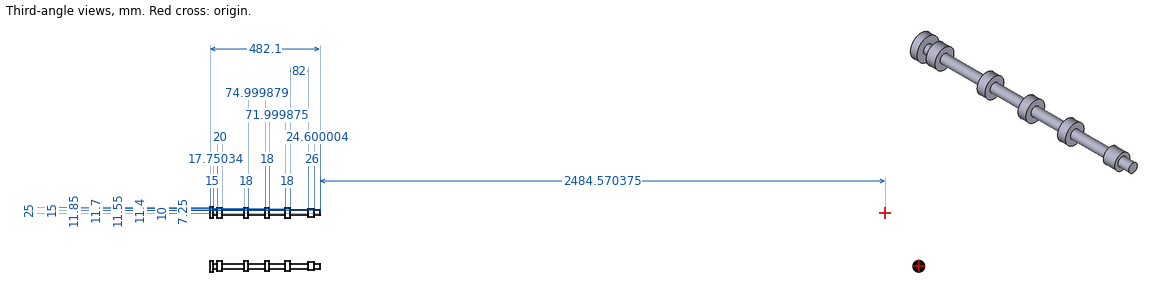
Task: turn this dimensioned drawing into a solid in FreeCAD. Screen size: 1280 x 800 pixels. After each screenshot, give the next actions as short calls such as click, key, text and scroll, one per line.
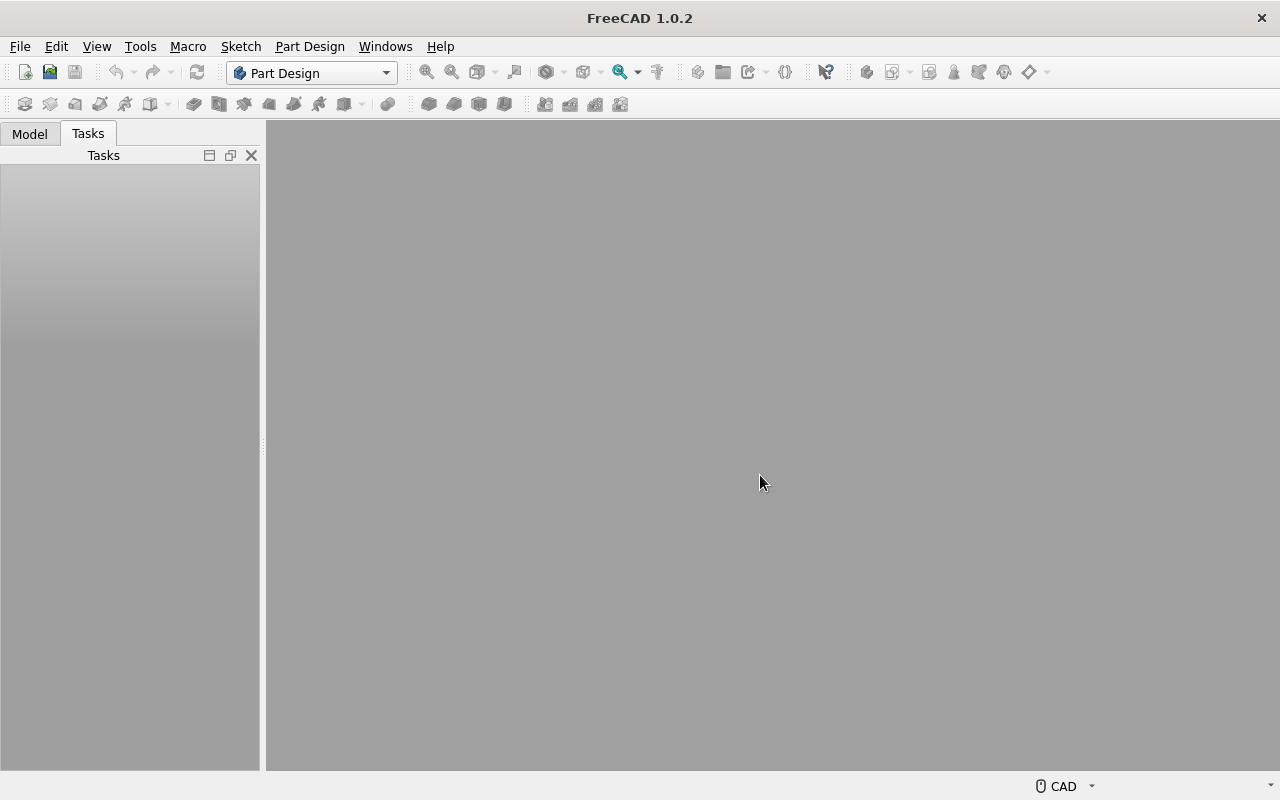
click(25, 72)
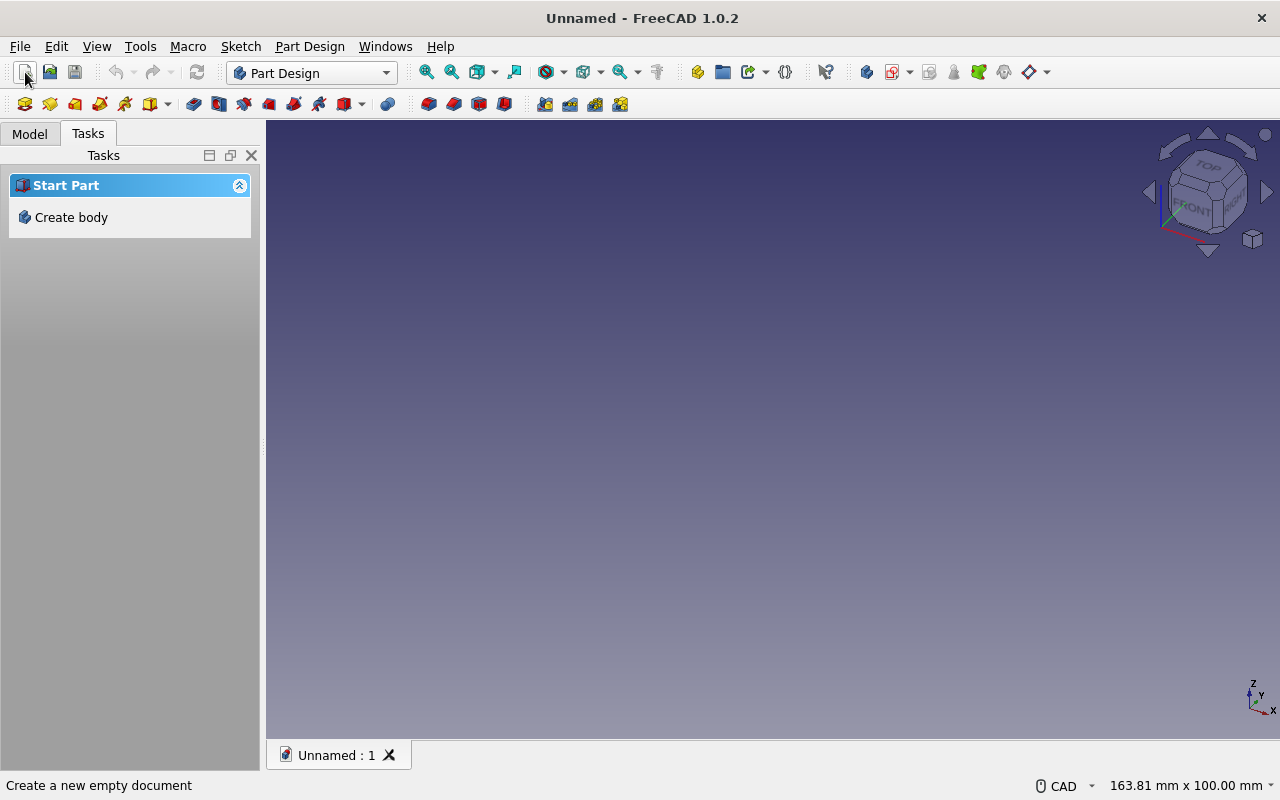
click(892, 72)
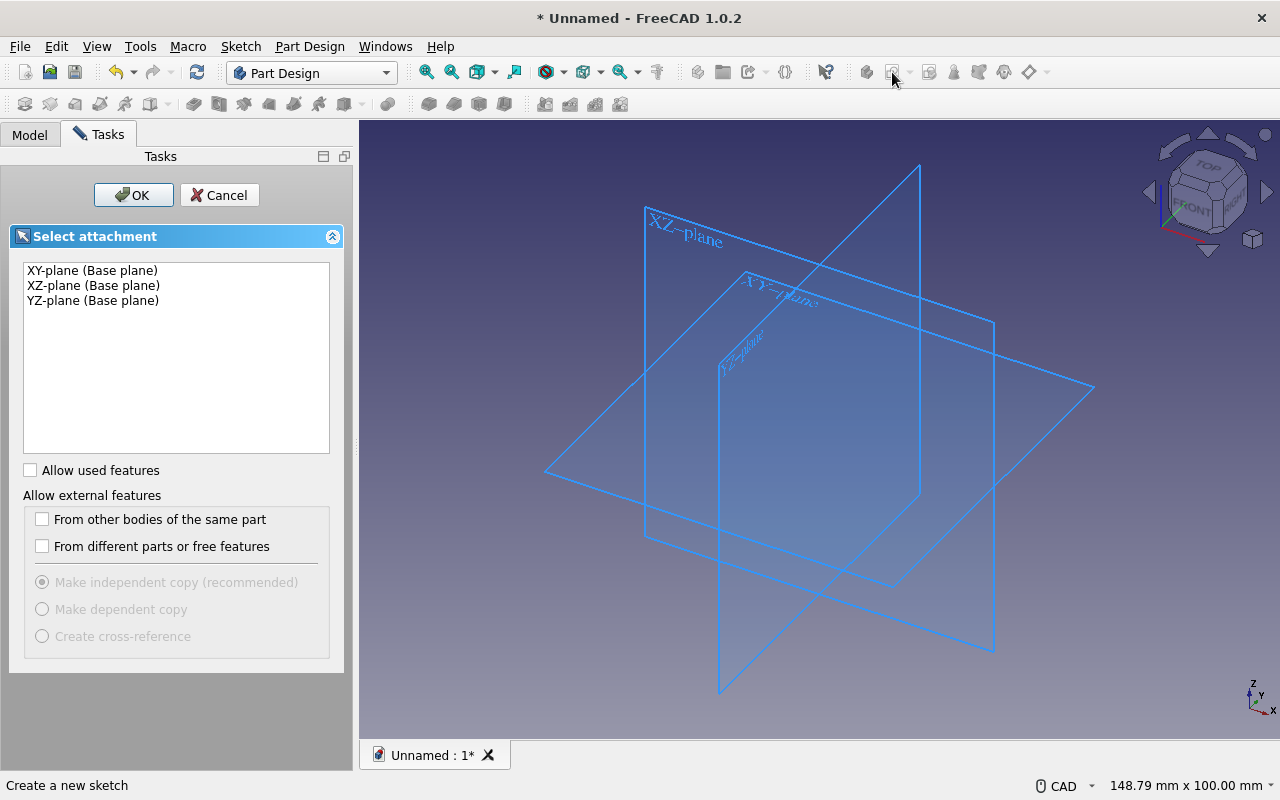
click(84, 270)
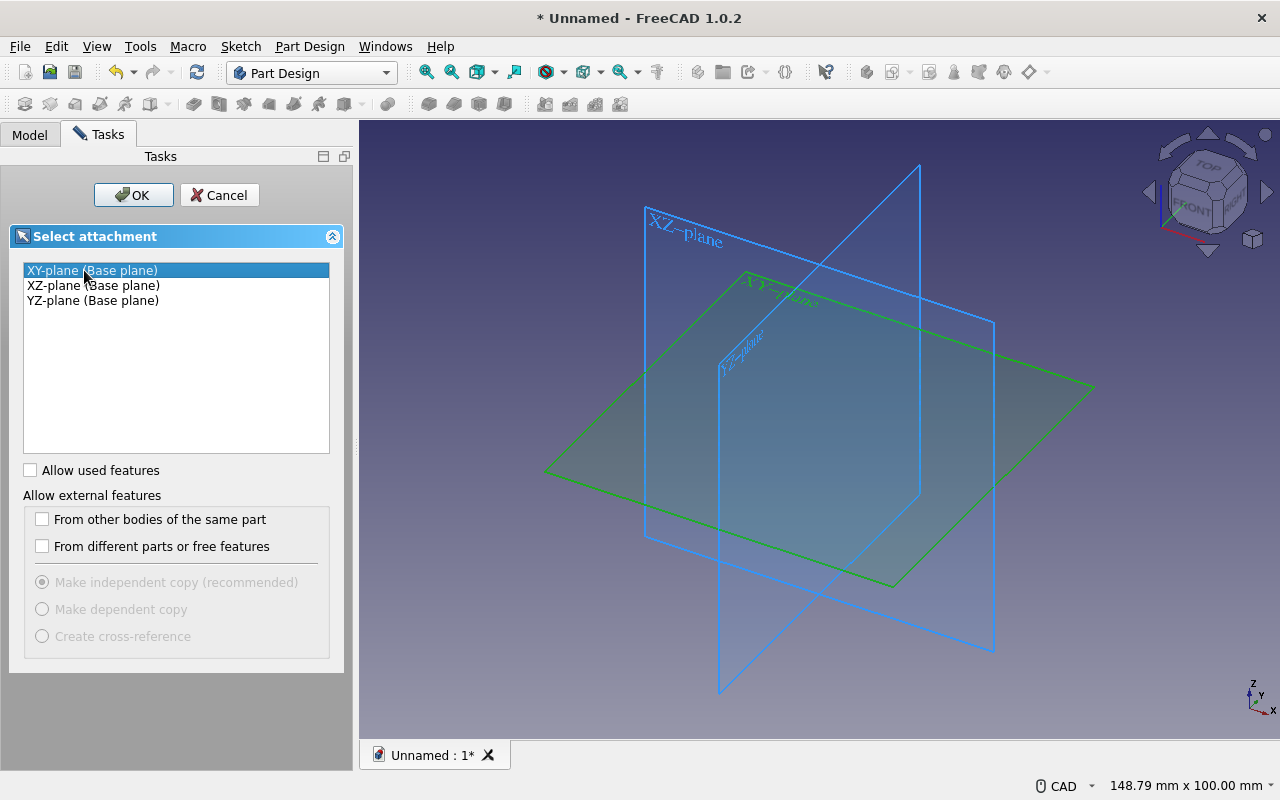
click(134, 195)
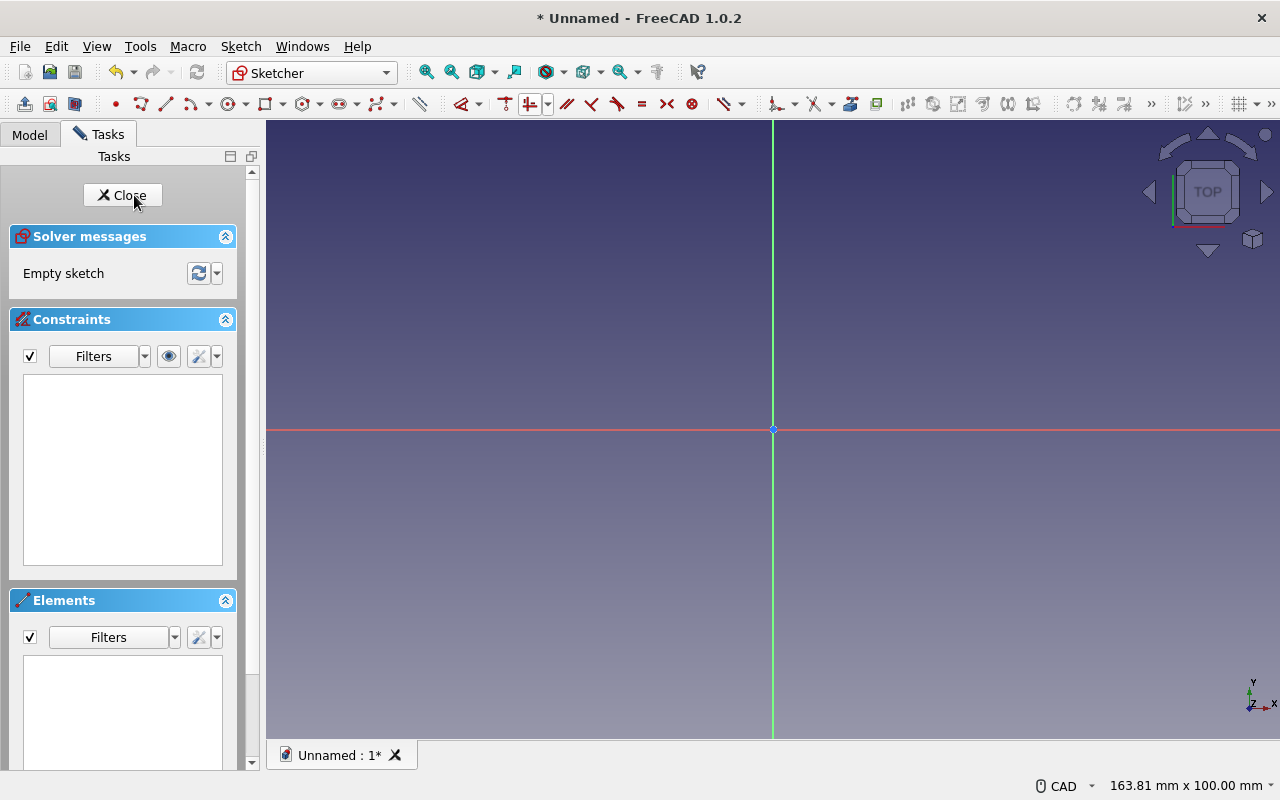
scroll(704, 430, down, 8)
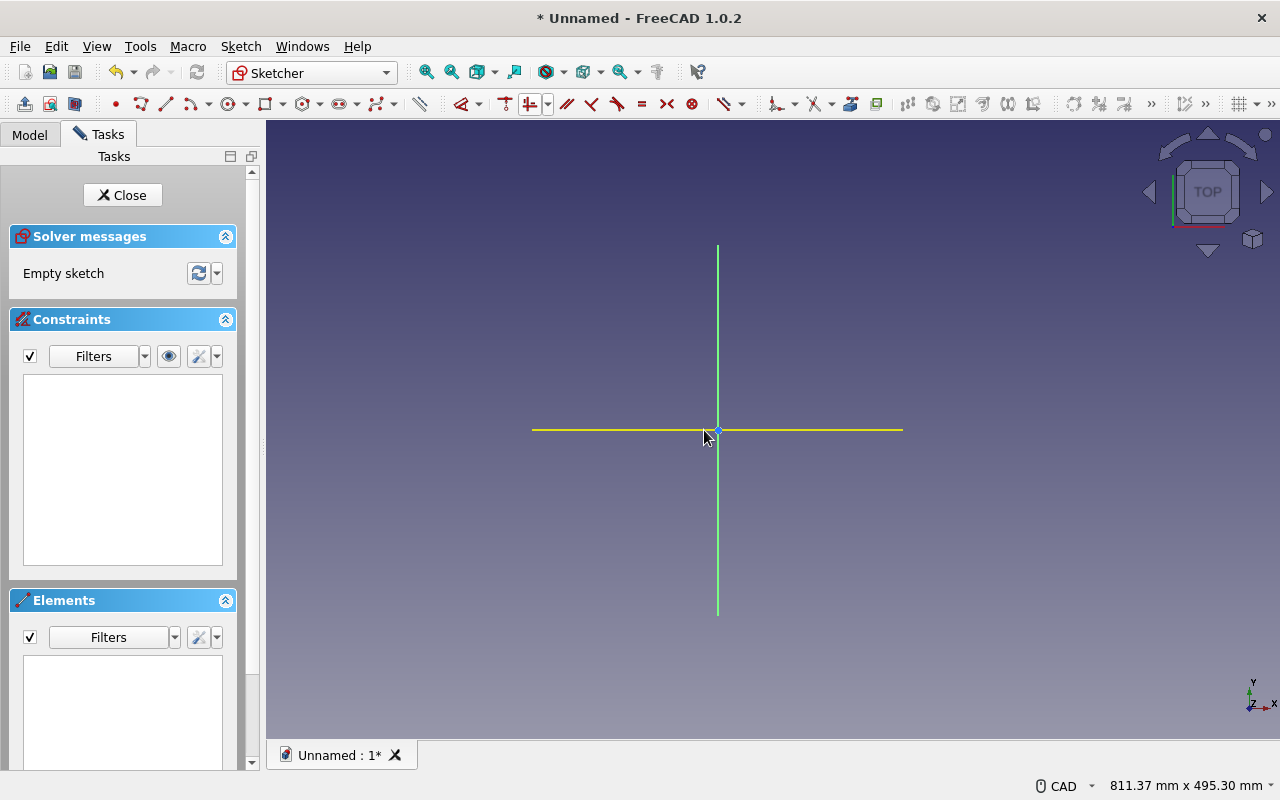
scroll(704, 430, down, 5)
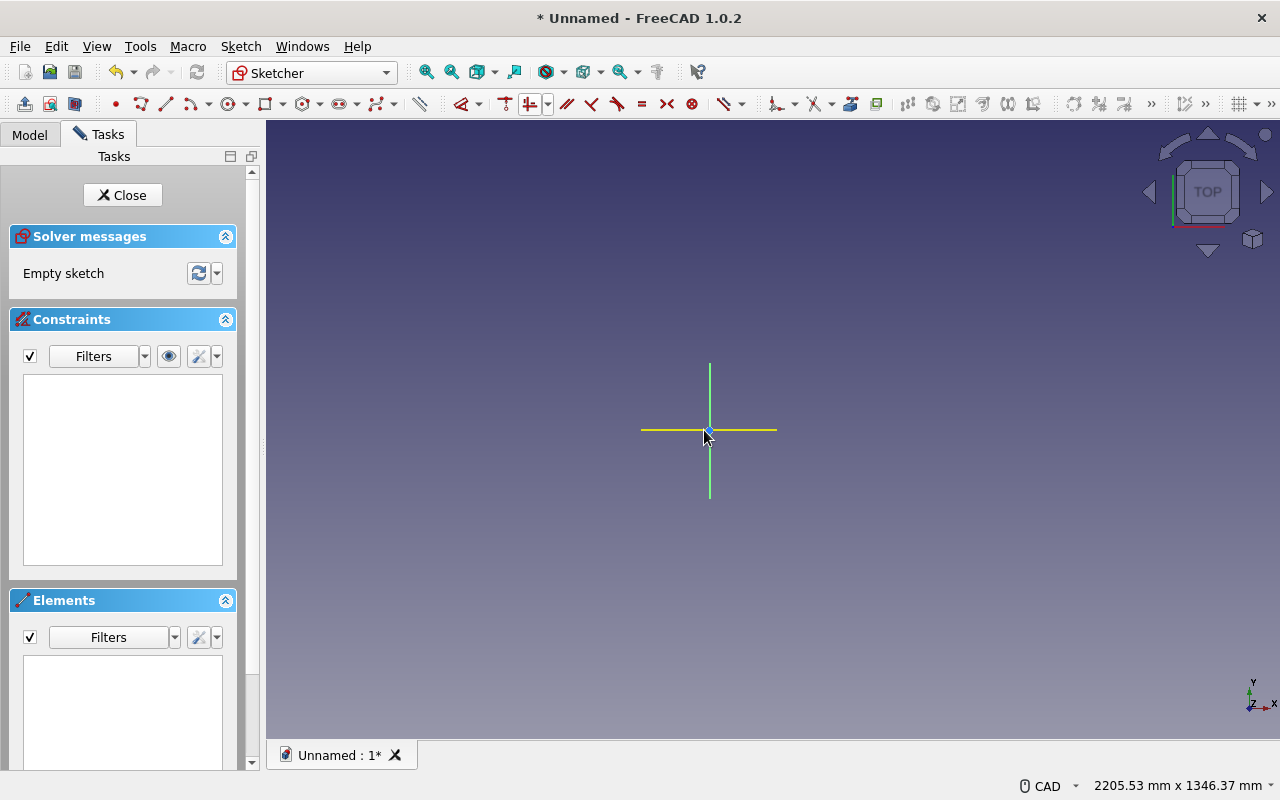
scroll(704, 430, down, 5)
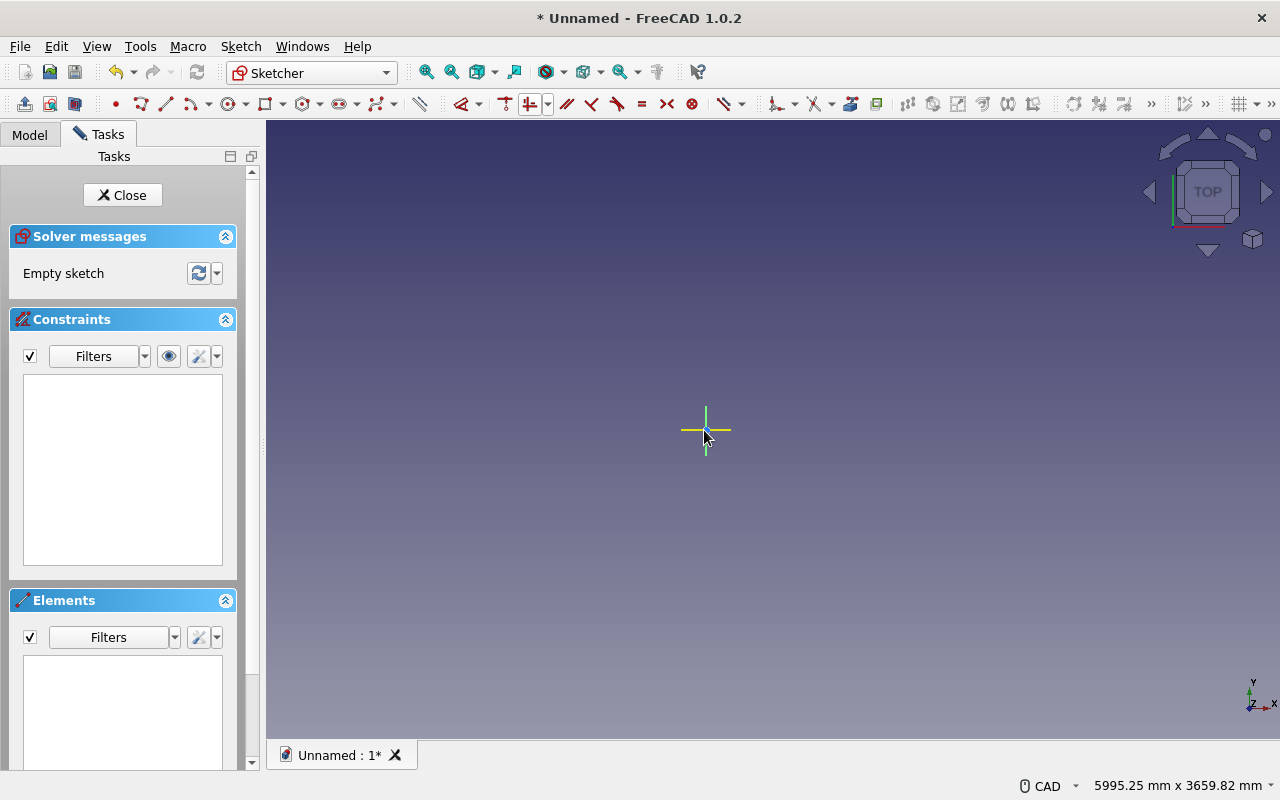
scroll(704, 430, down, 5)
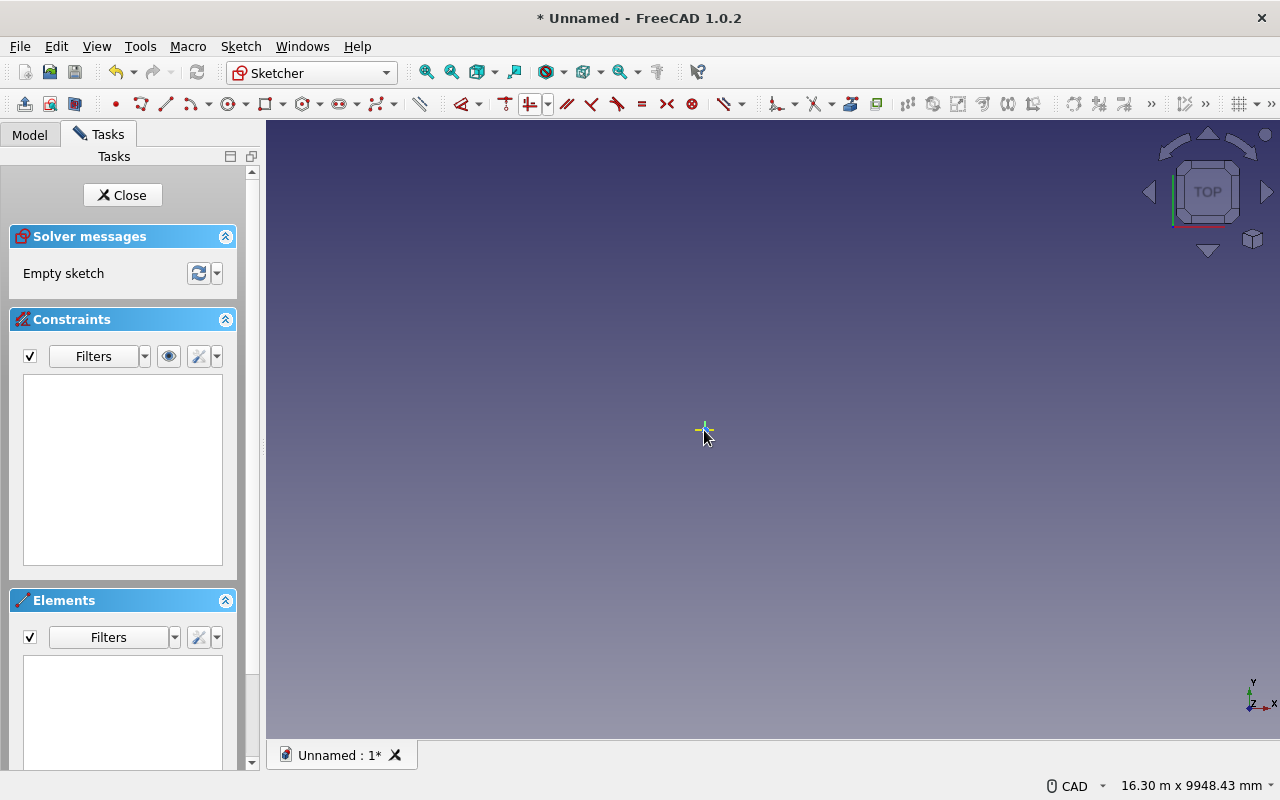
scroll(527, 430, up, 15)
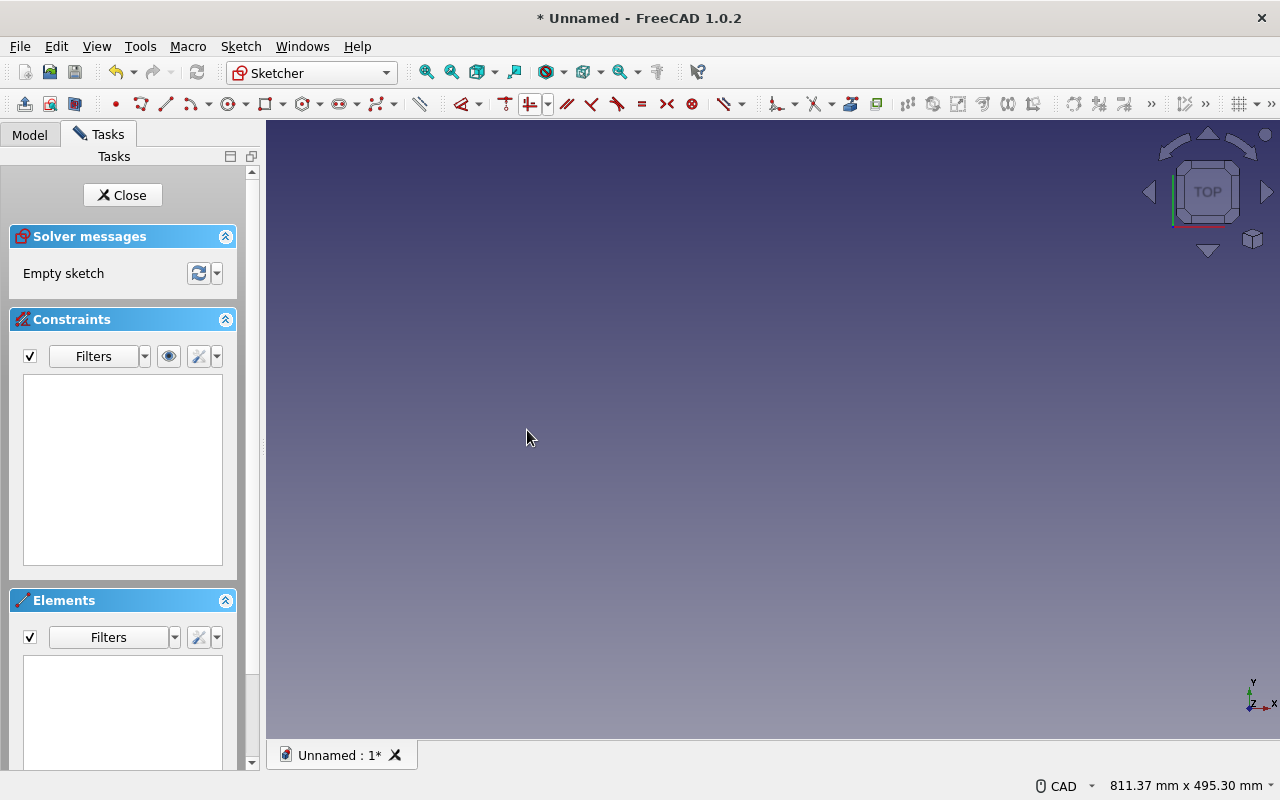
click(141, 104)